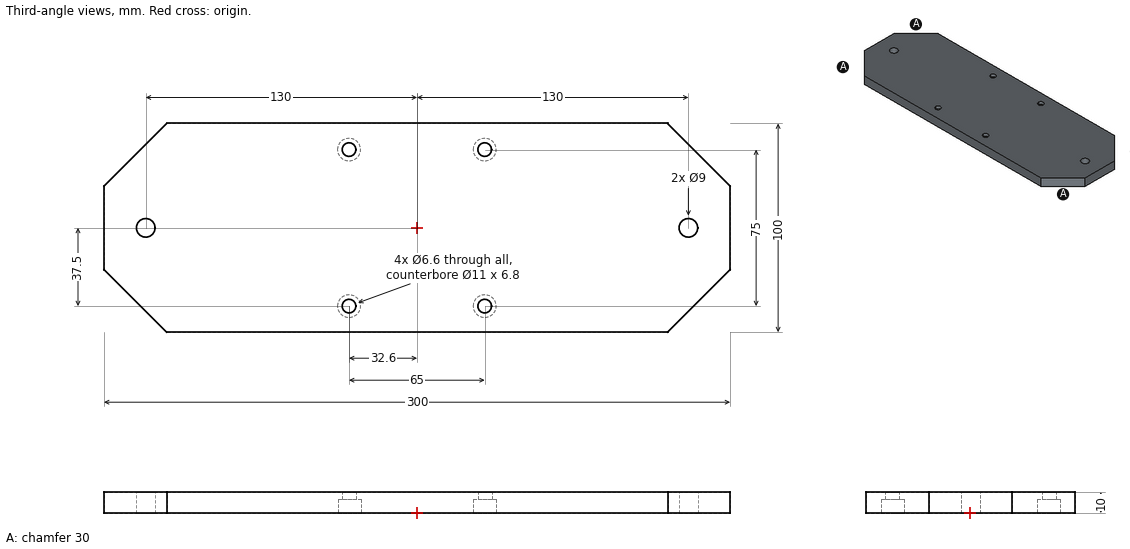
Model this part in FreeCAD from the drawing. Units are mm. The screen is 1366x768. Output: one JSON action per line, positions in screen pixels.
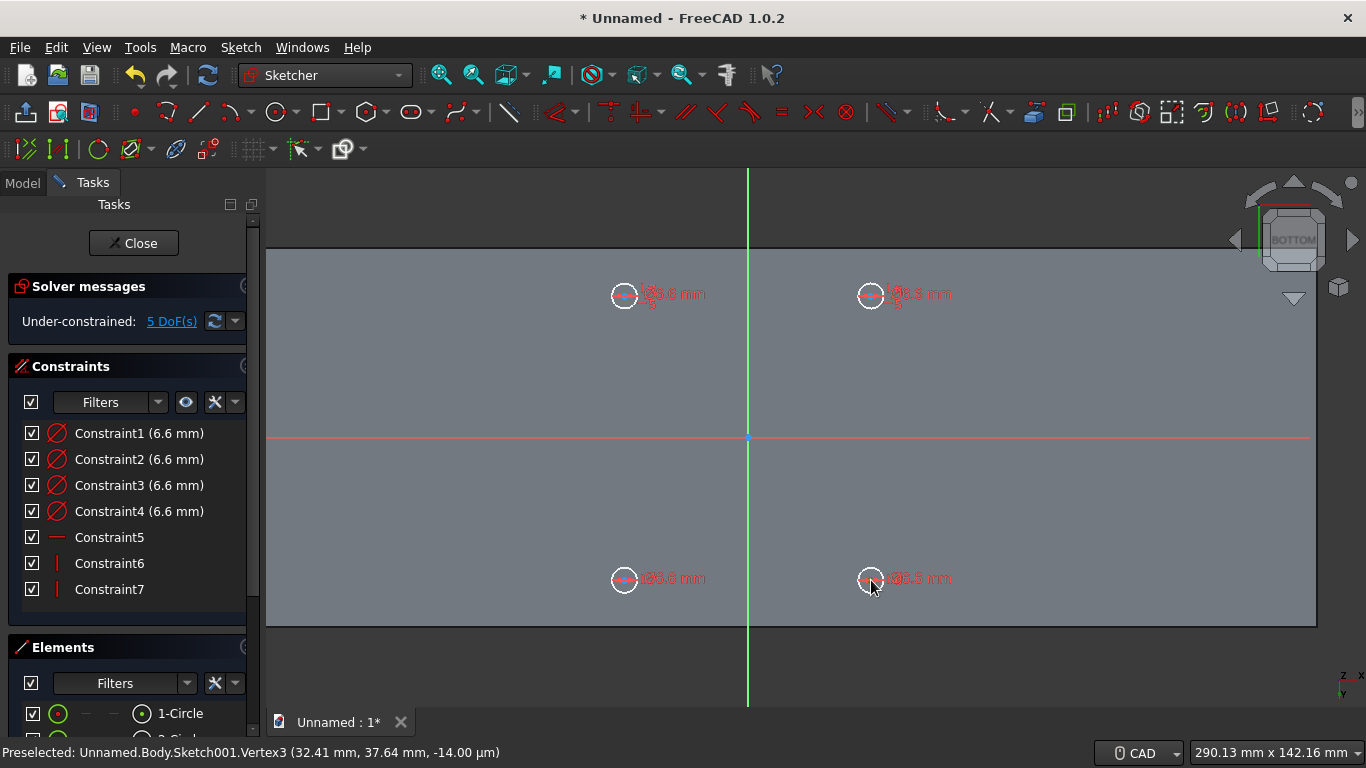
{"action": "left_click", "coordinate": [625, 580]}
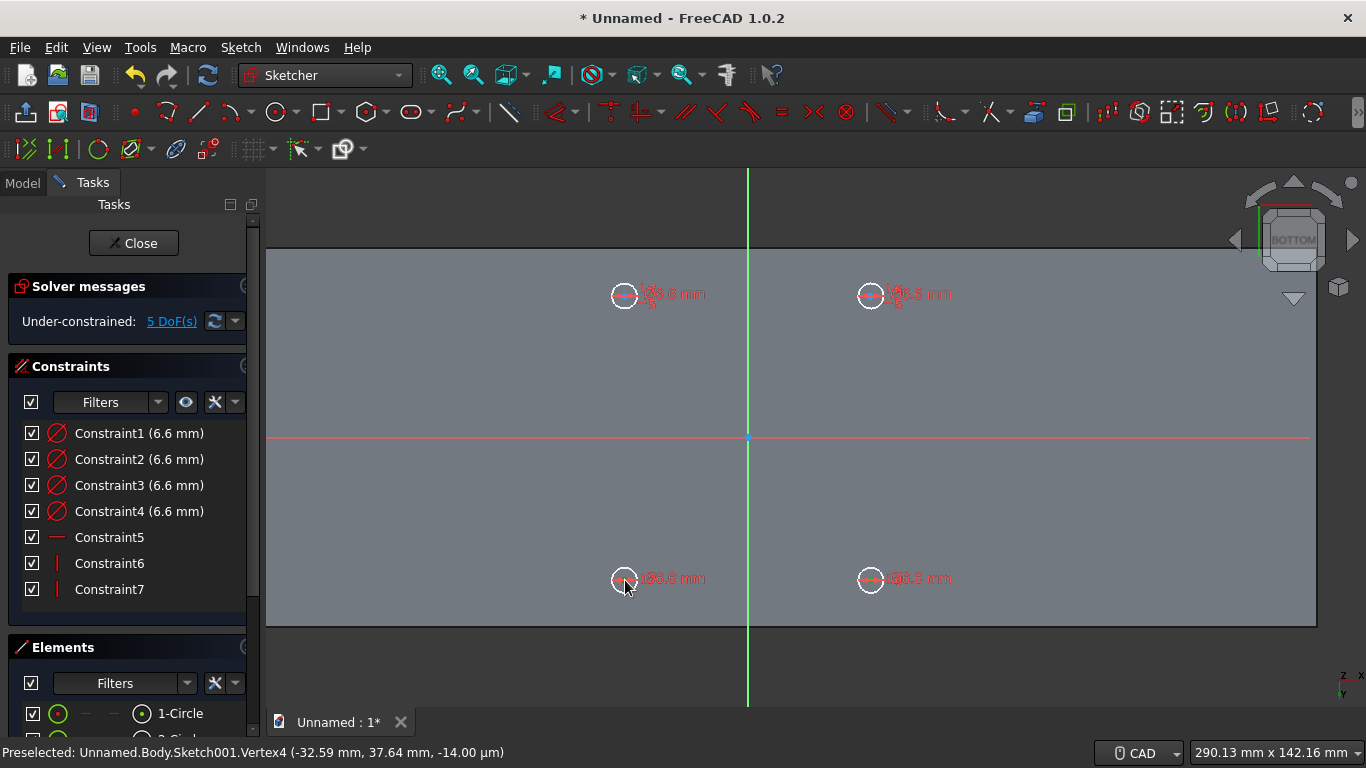
{"action": "key", "text": "h"}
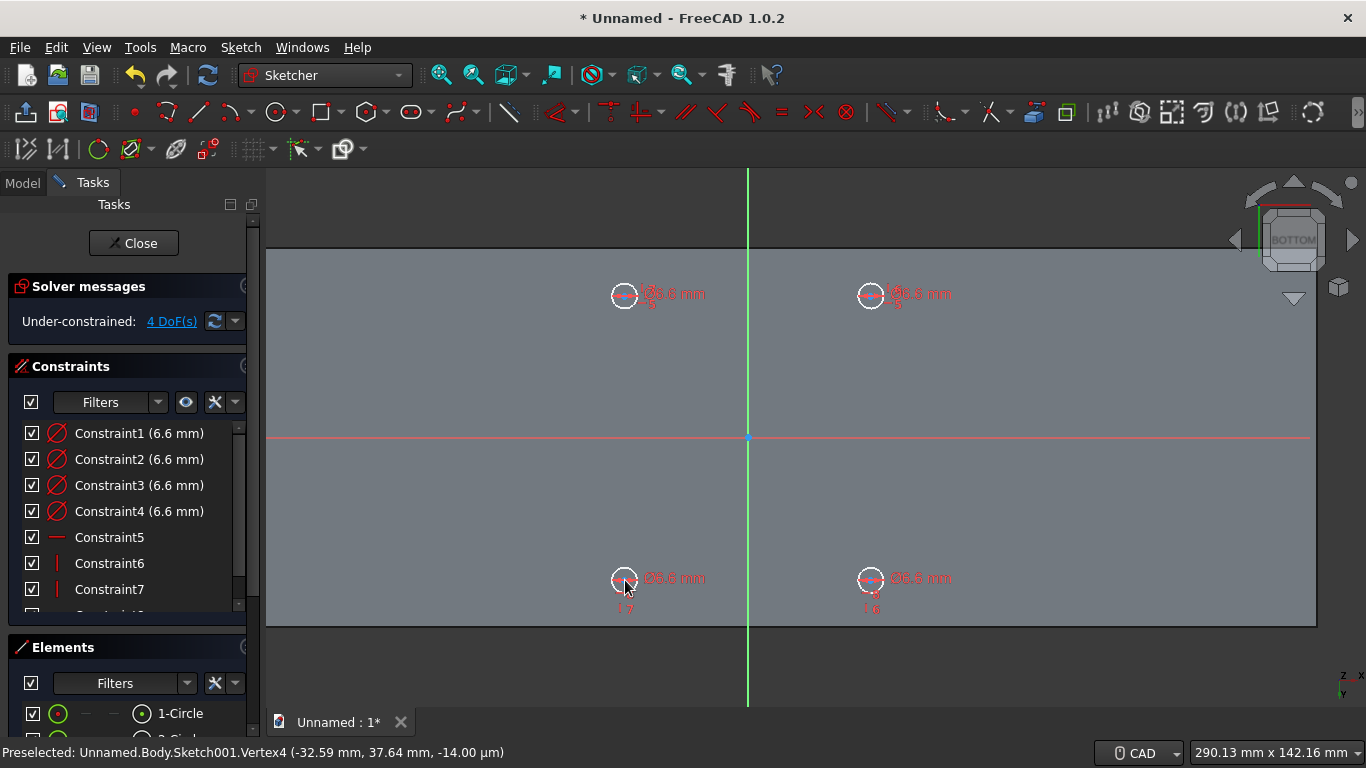
{"action": "left_click", "coordinate": [625, 296]}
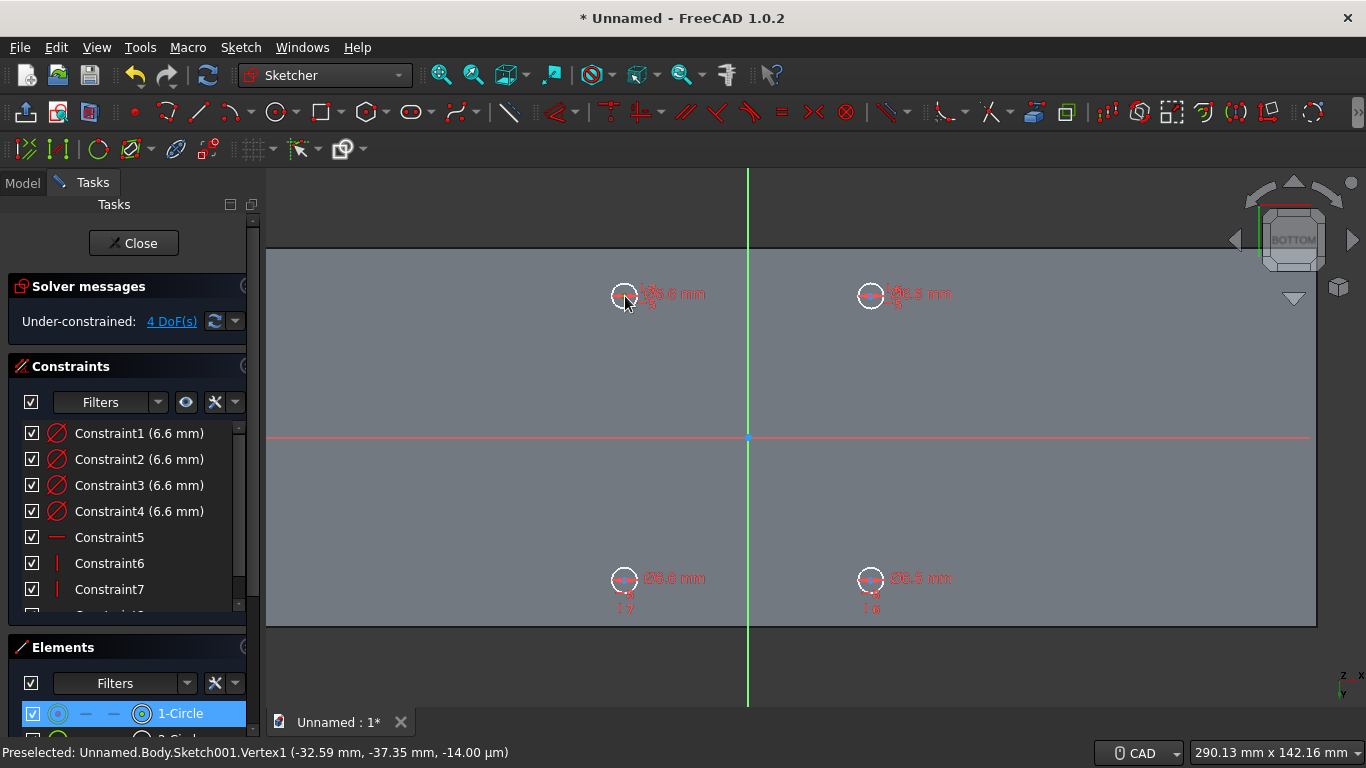
{"action": "left_click", "coordinate": [871, 296]}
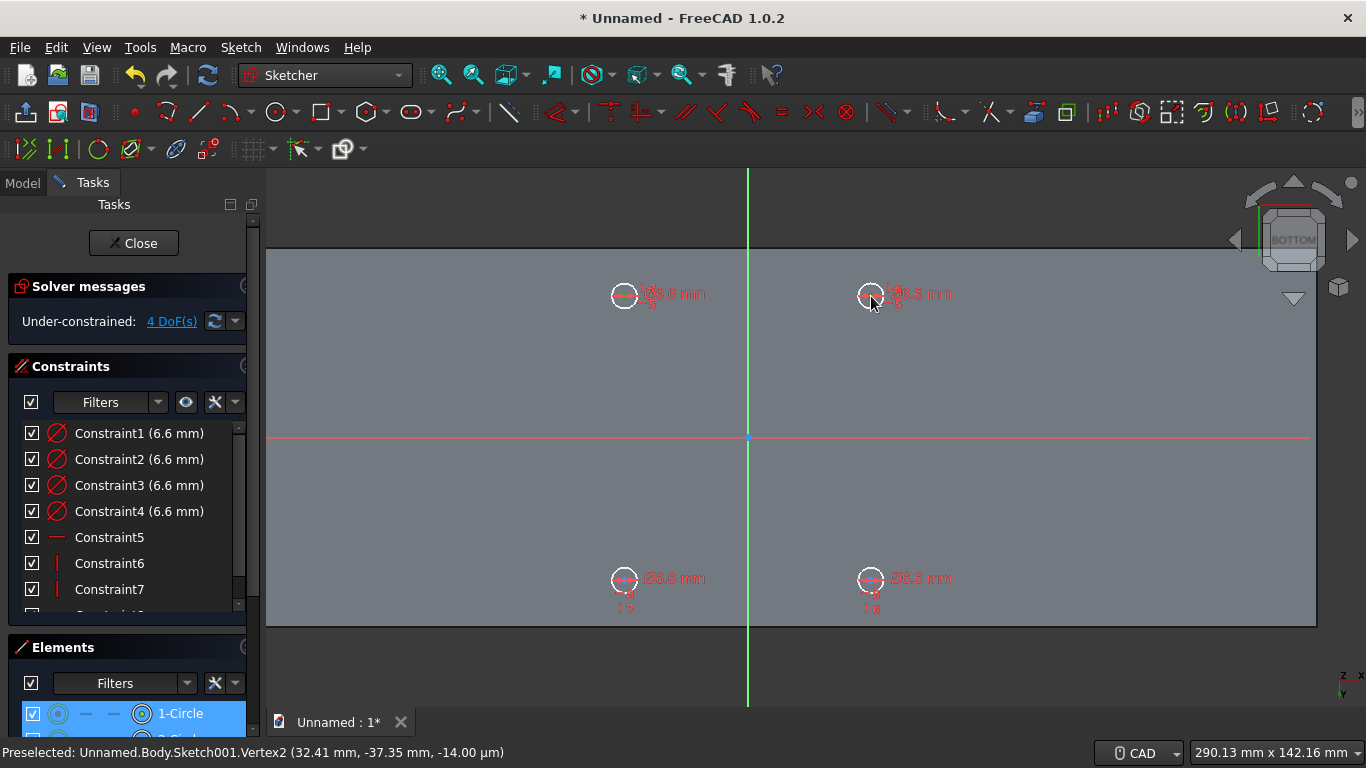
{"action": "left_click", "coordinate": [578, 112]}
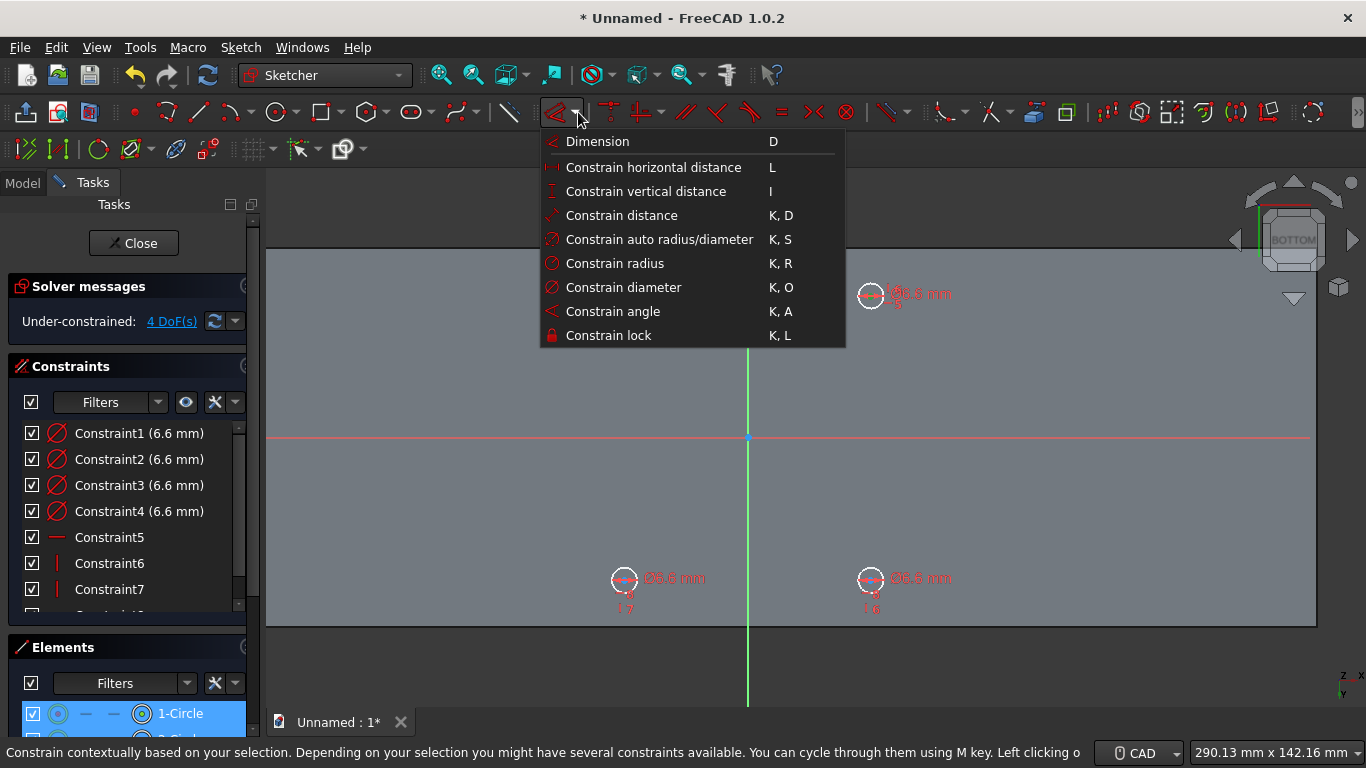
{"action": "left_click", "coordinate": [693, 167]}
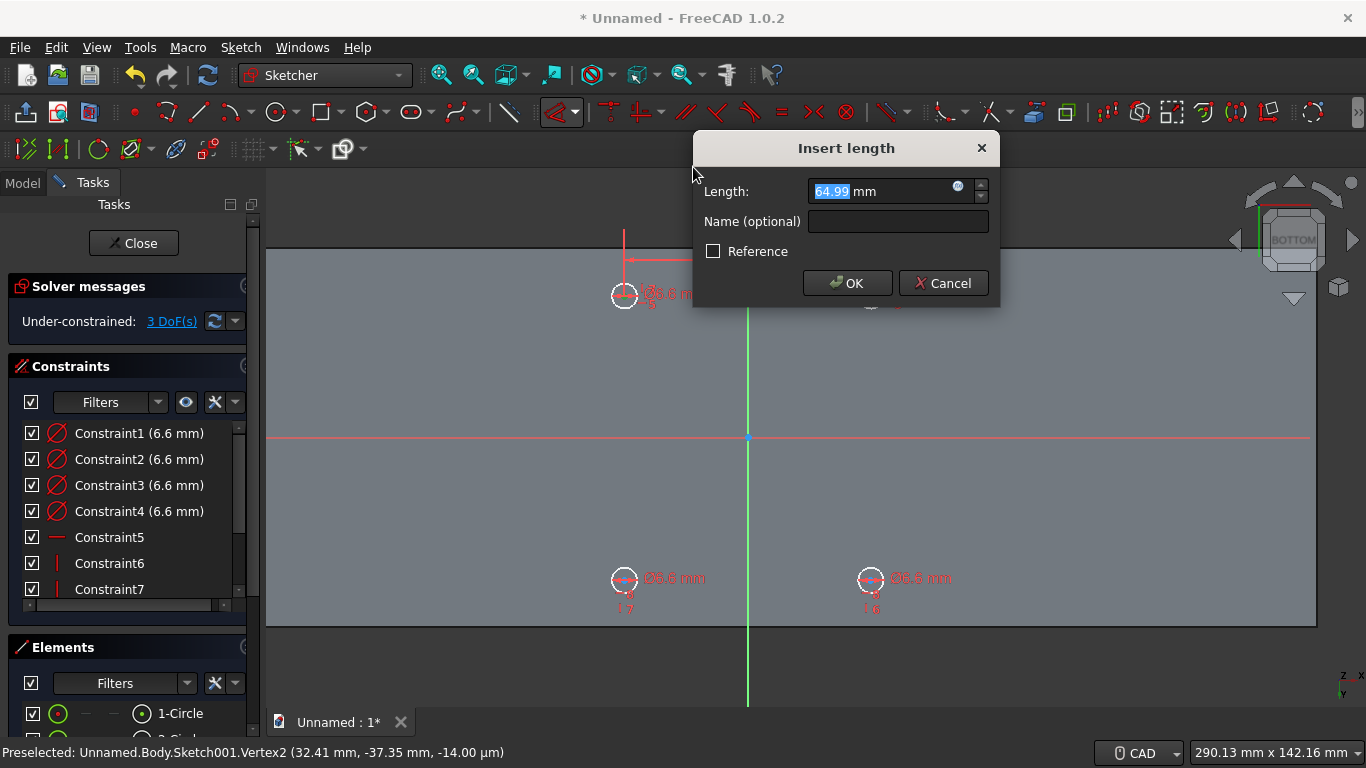
{"action": "type", "text": "65"}
{"action": "key", "text": "Return"}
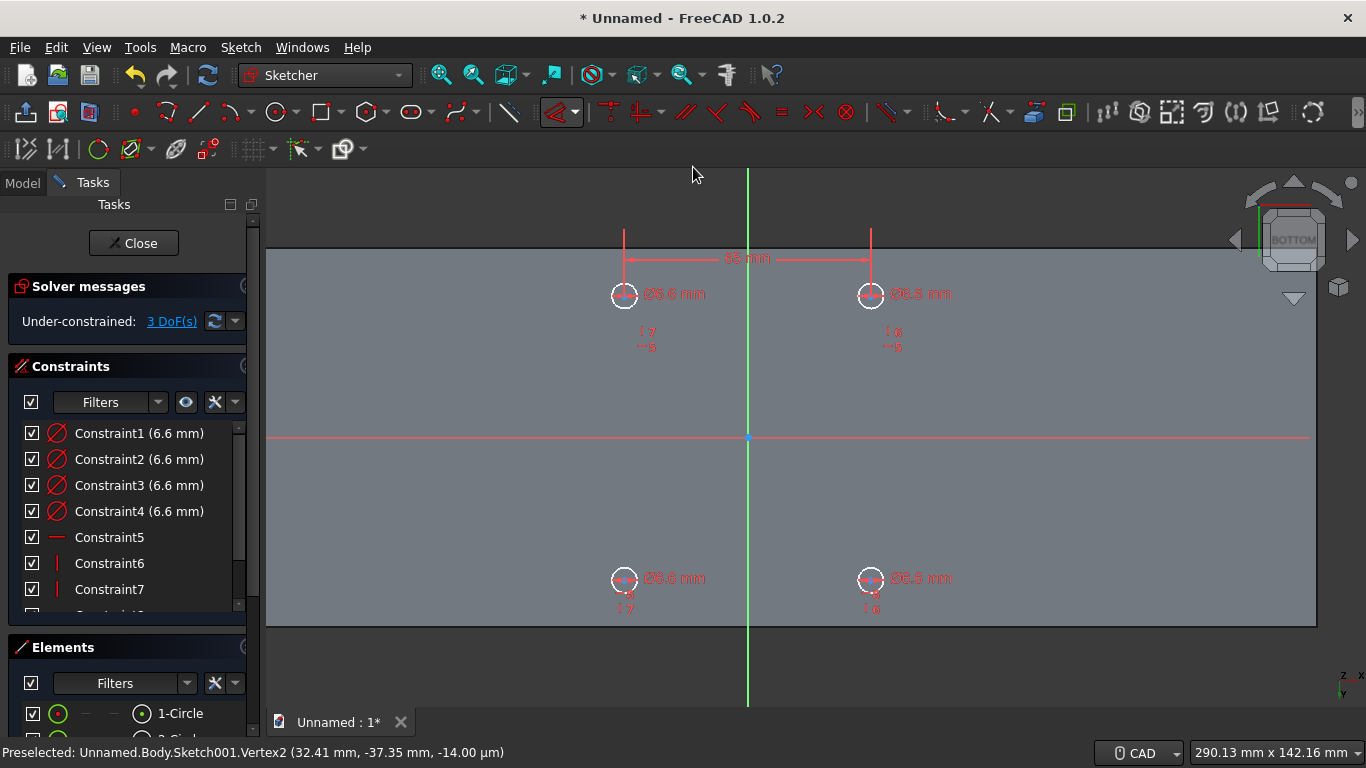
{"action": "left_click", "coordinate": [871, 296]}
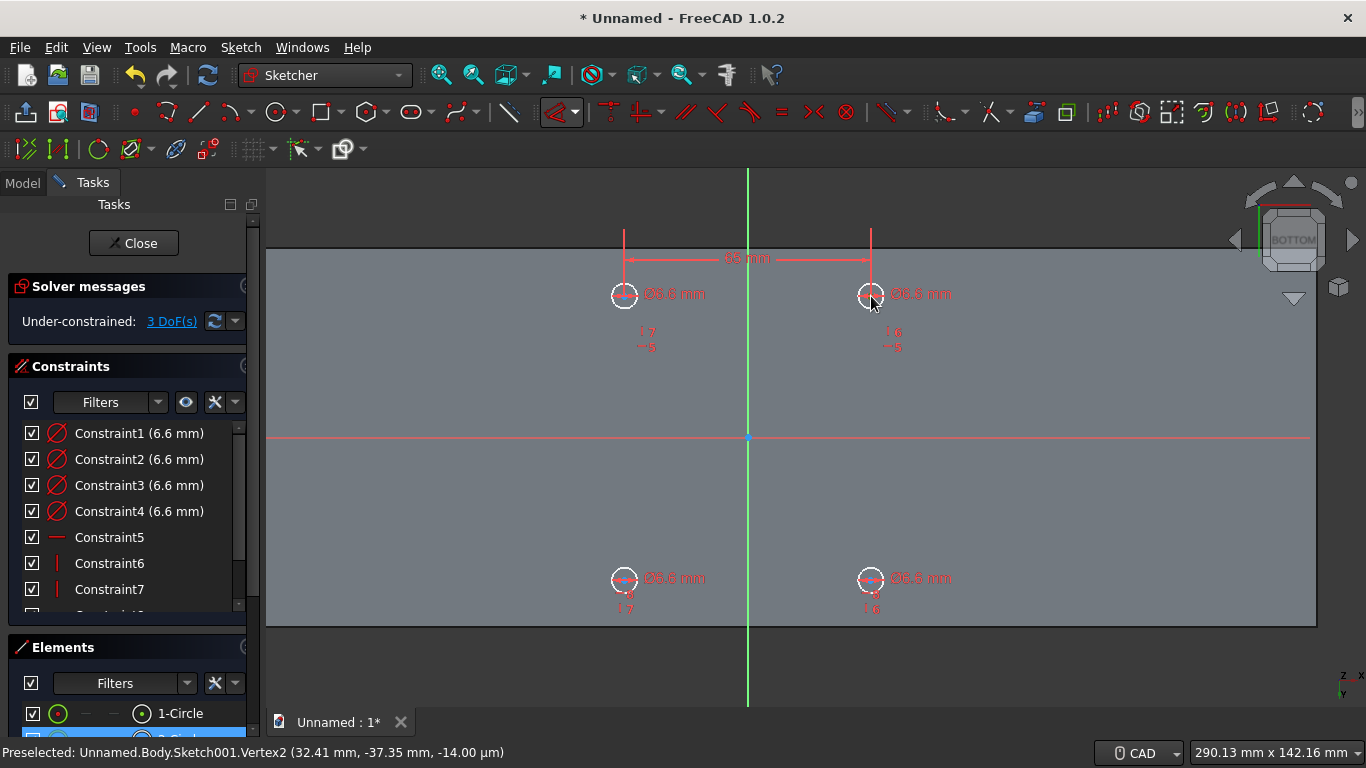
{"action": "left_click", "coordinate": [871, 580]}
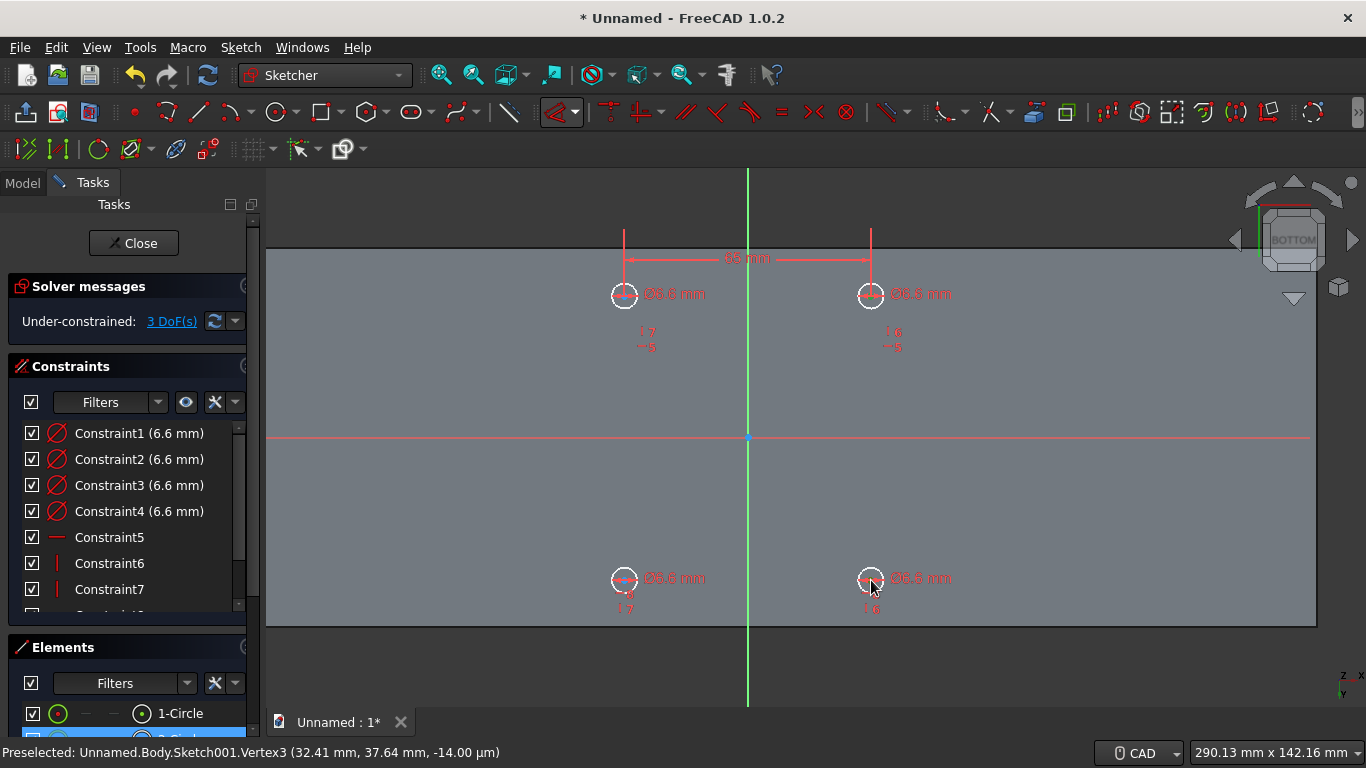
{"action": "key", "text": "i"}